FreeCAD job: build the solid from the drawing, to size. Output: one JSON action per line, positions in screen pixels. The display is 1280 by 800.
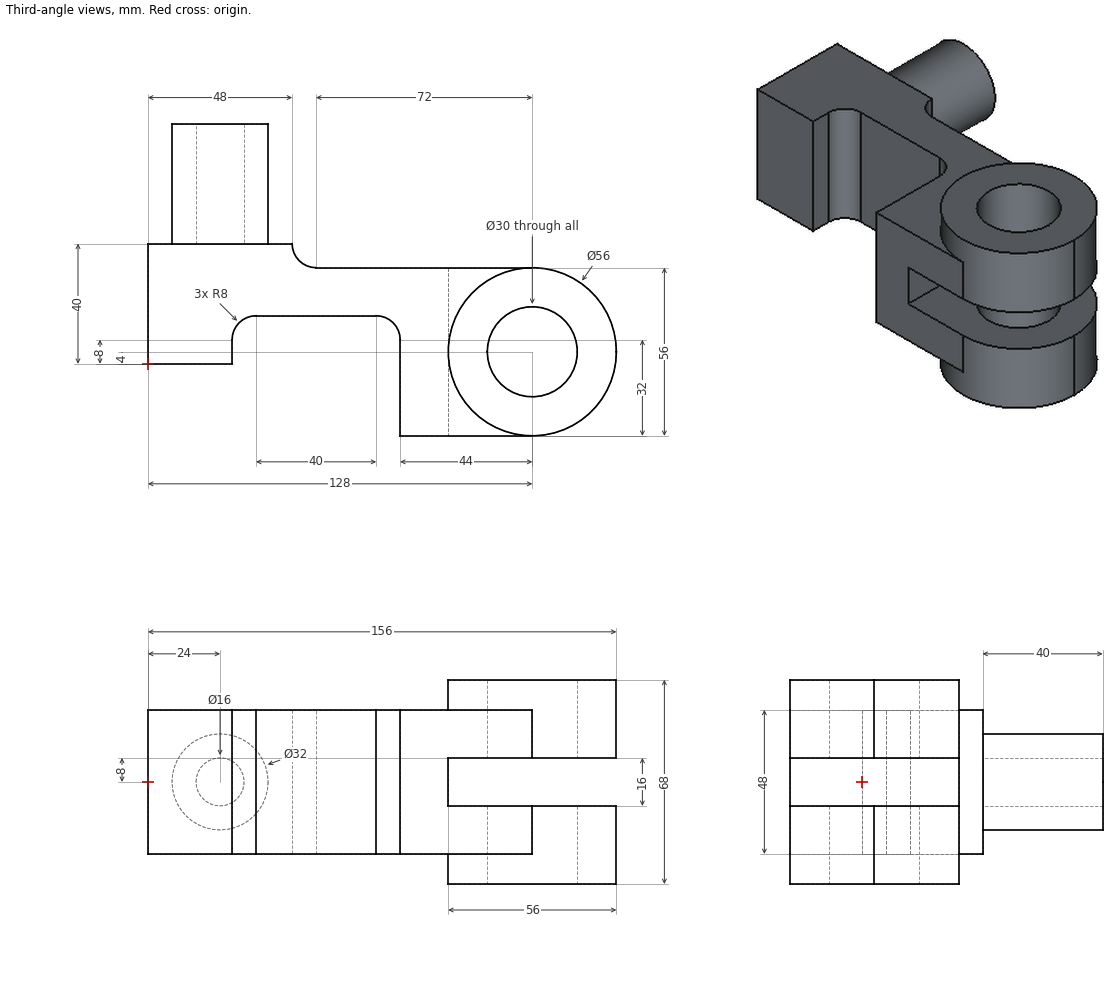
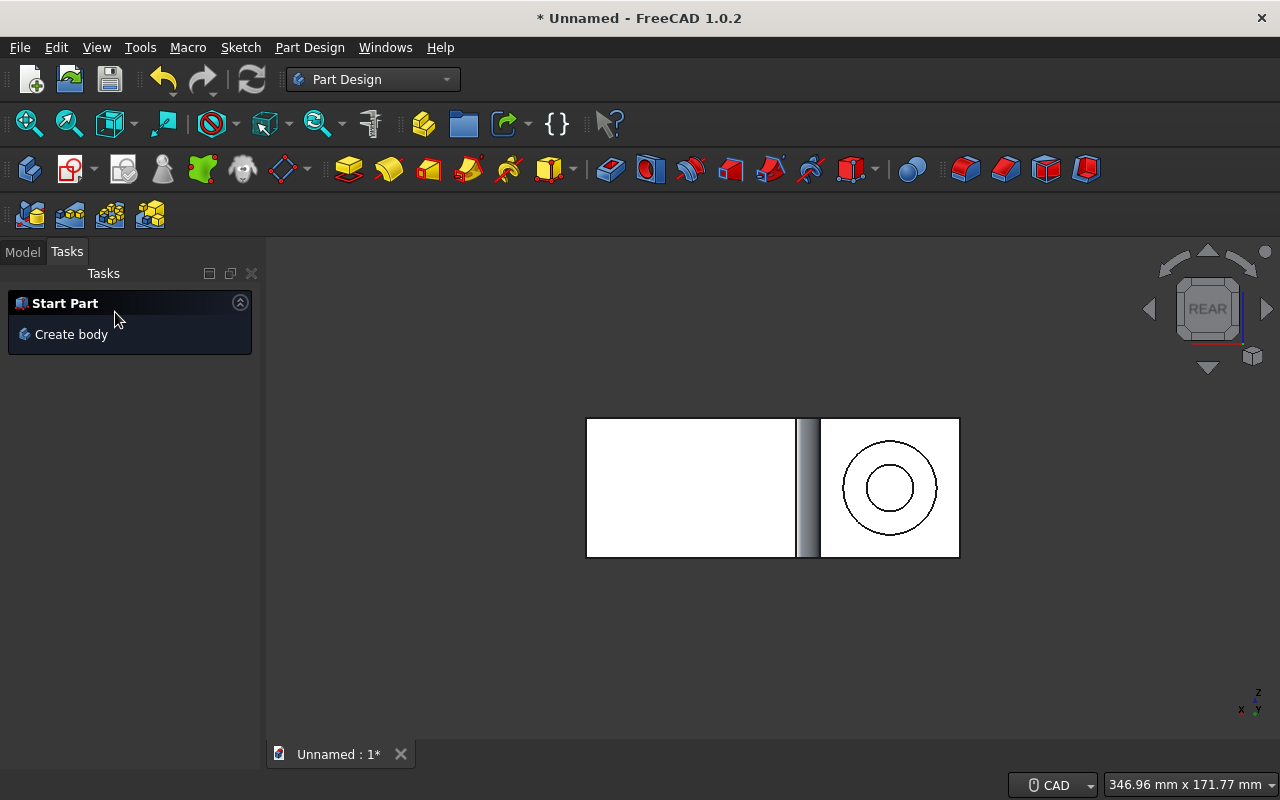
{"action": "left_click", "coordinate": [70, 170]}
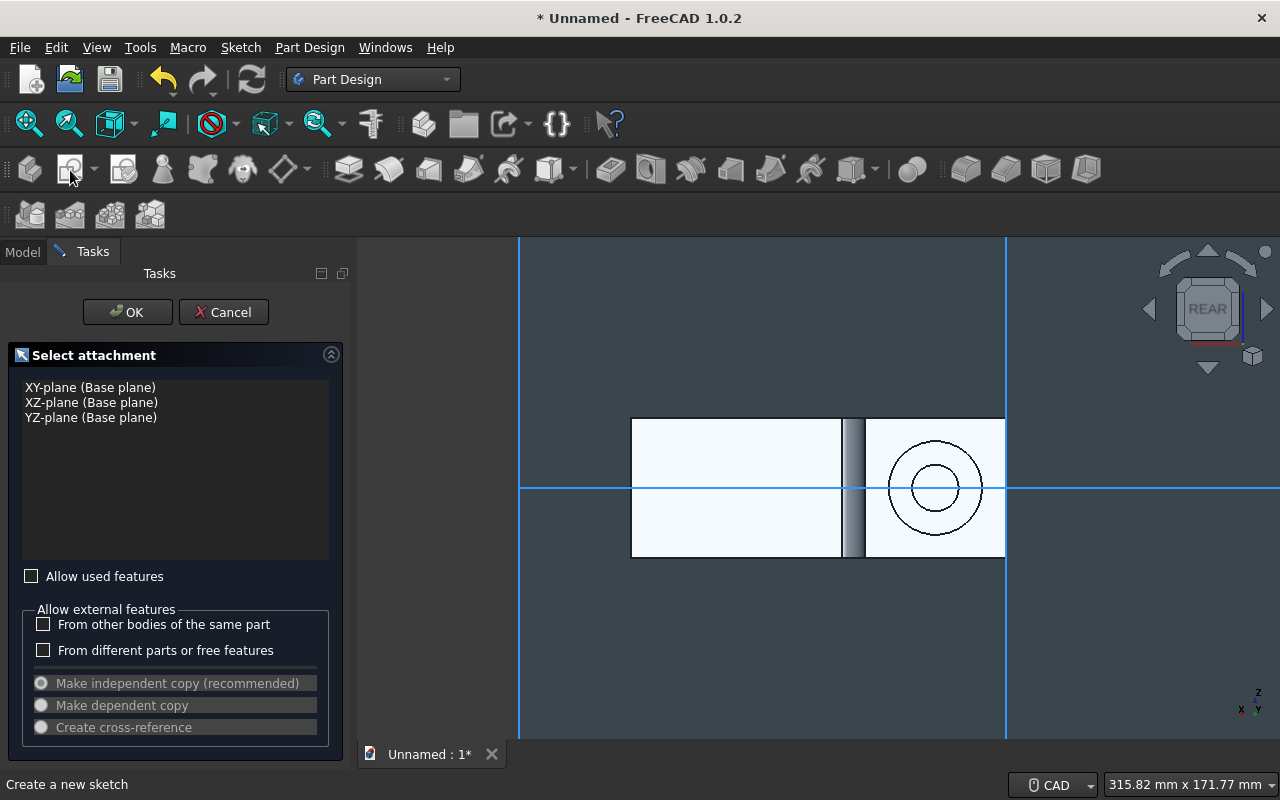
{"action": "left_click", "coordinate": [82, 388]}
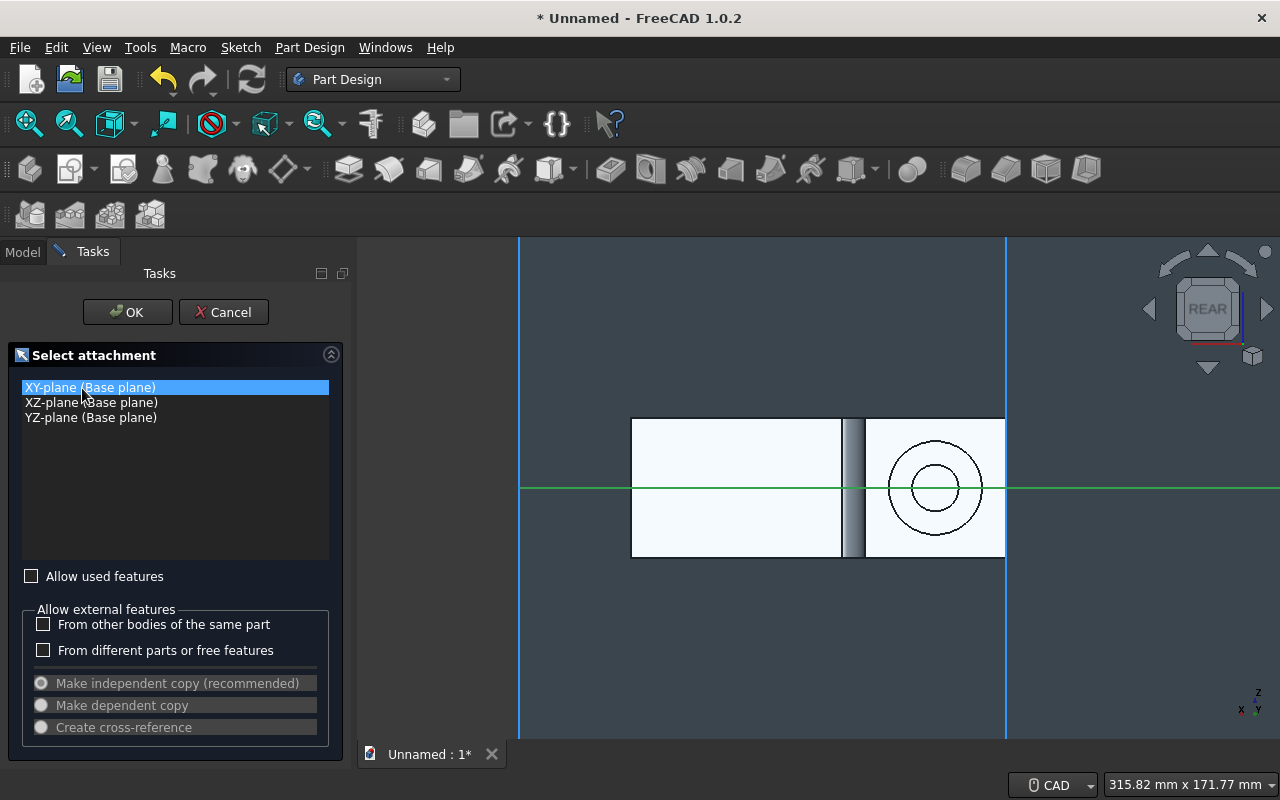
{"action": "left_click", "coordinate": [128, 312]}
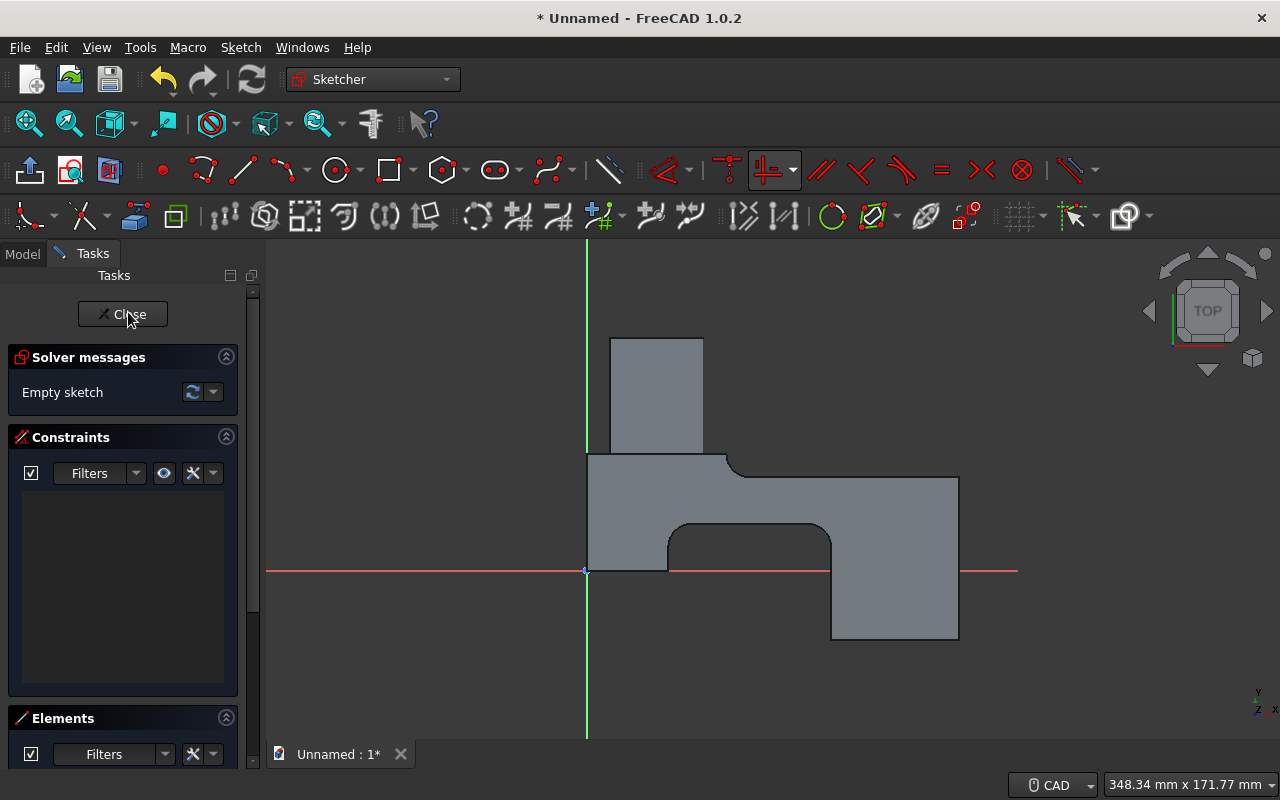
{"action": "key", "text": "q s"}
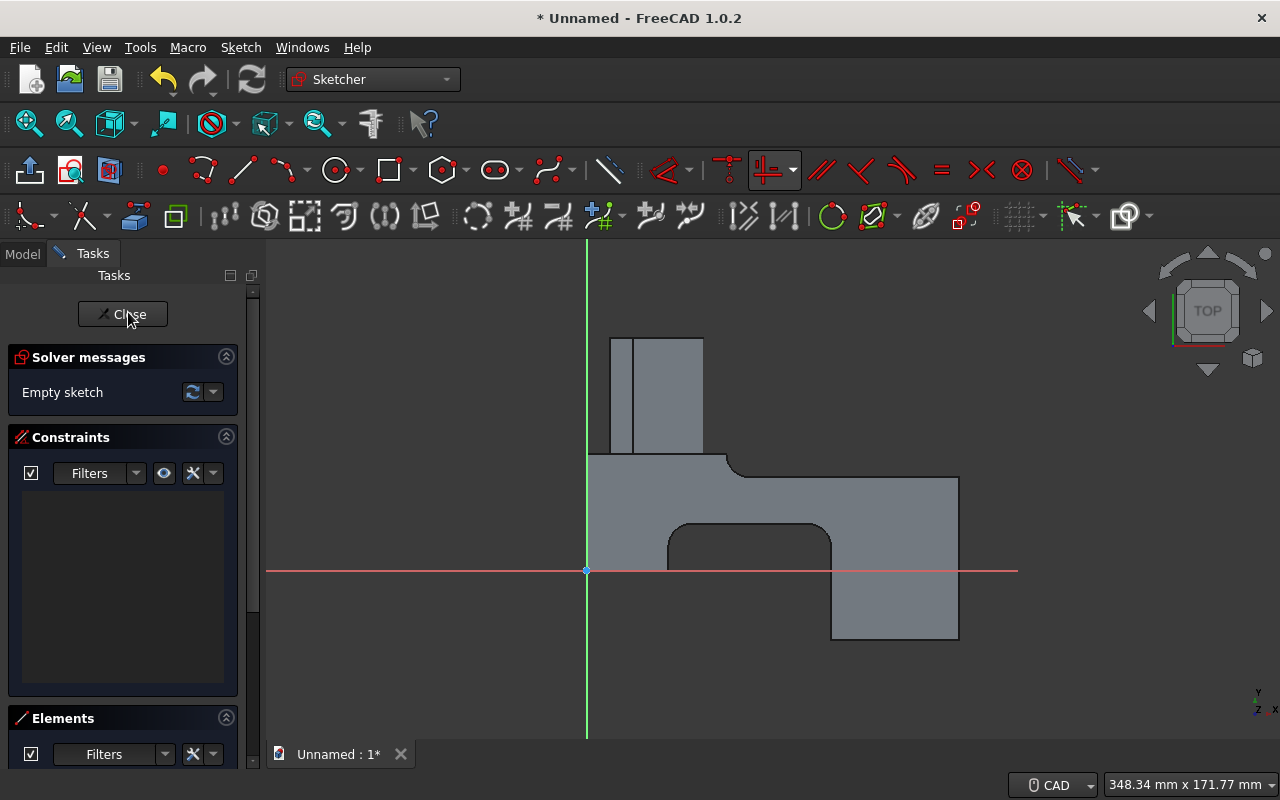
{"action": "scroll", "coordinate": [1115, 644], "scroll_direction": "up", "scroll_amount": 3}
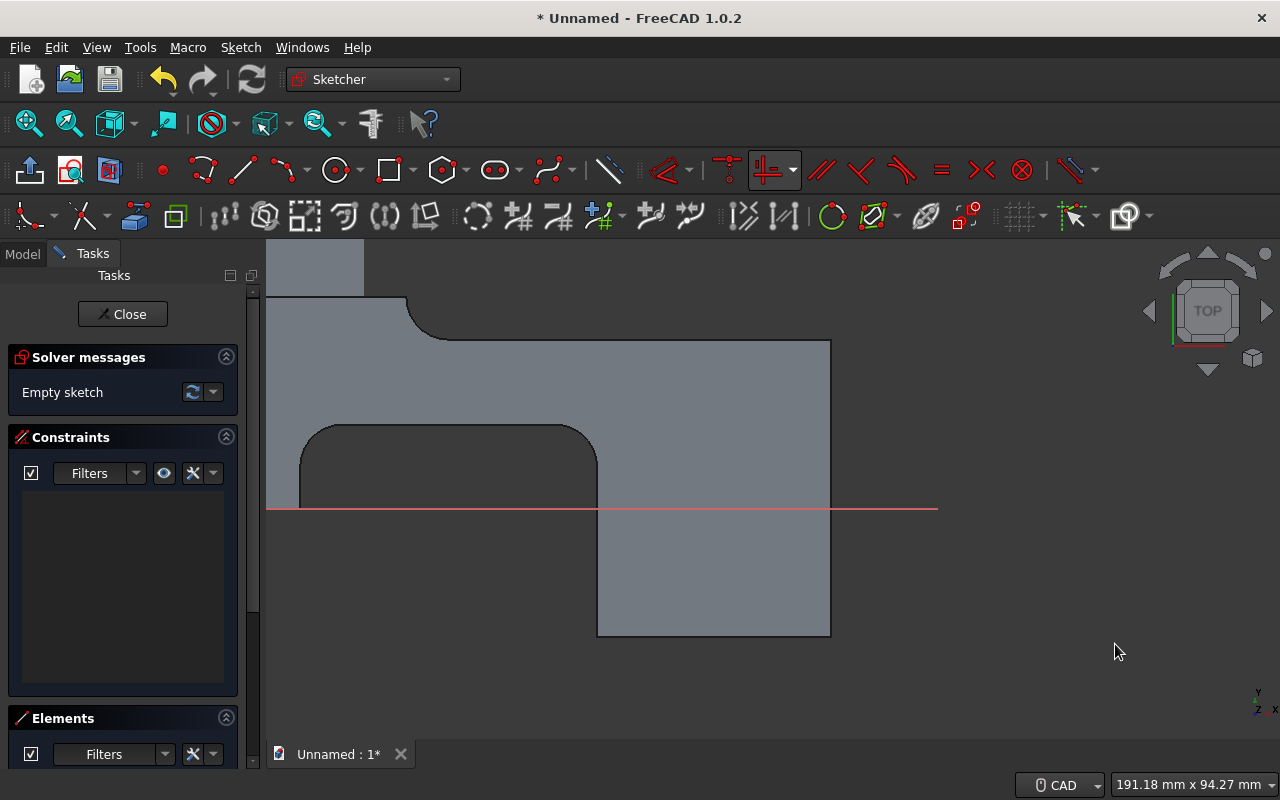
{"action": "key", "text": "g c"}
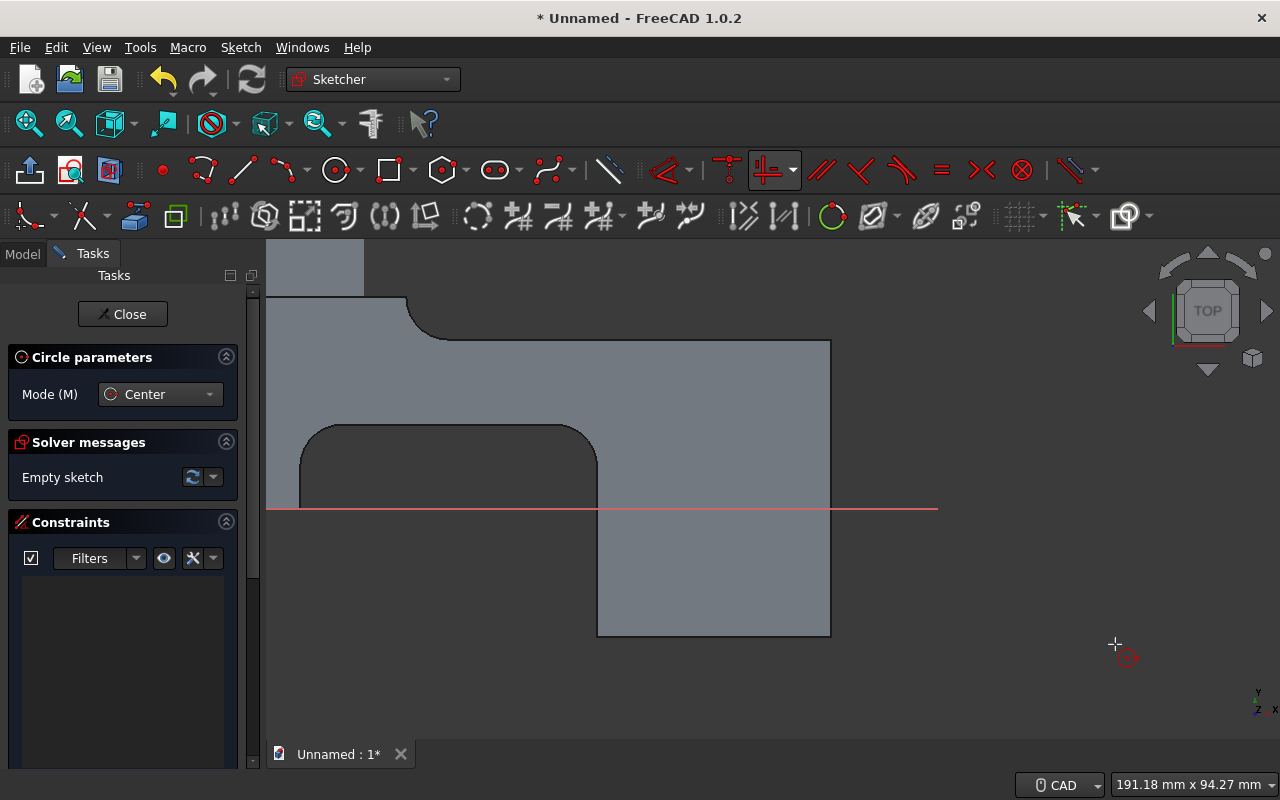
{"action": "left_click", "coordinate": [831, 488]}
{"action": "mouse_move", "coordinate": [936, 383]}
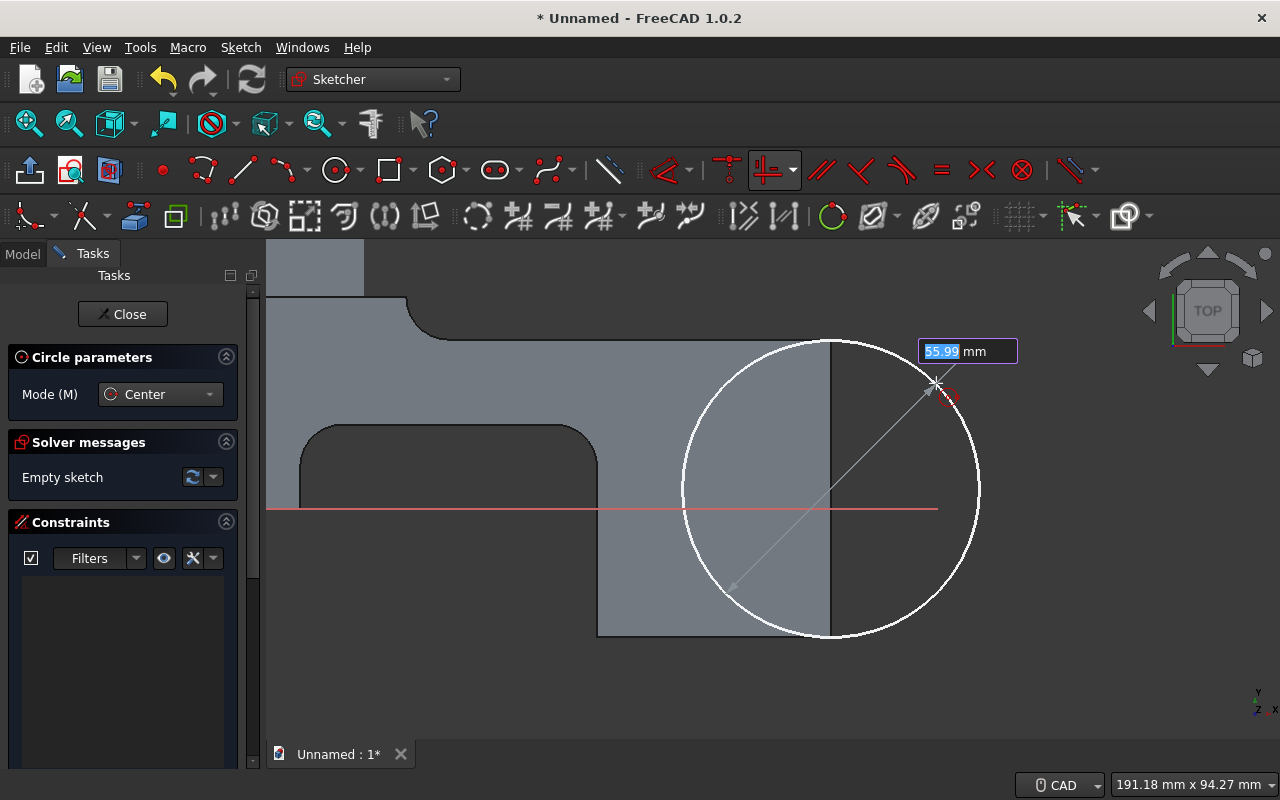
{"action": "type", "text": "56"}
{"action": "key", "text": "Return"}
{"action": "key", "text": "Escape"}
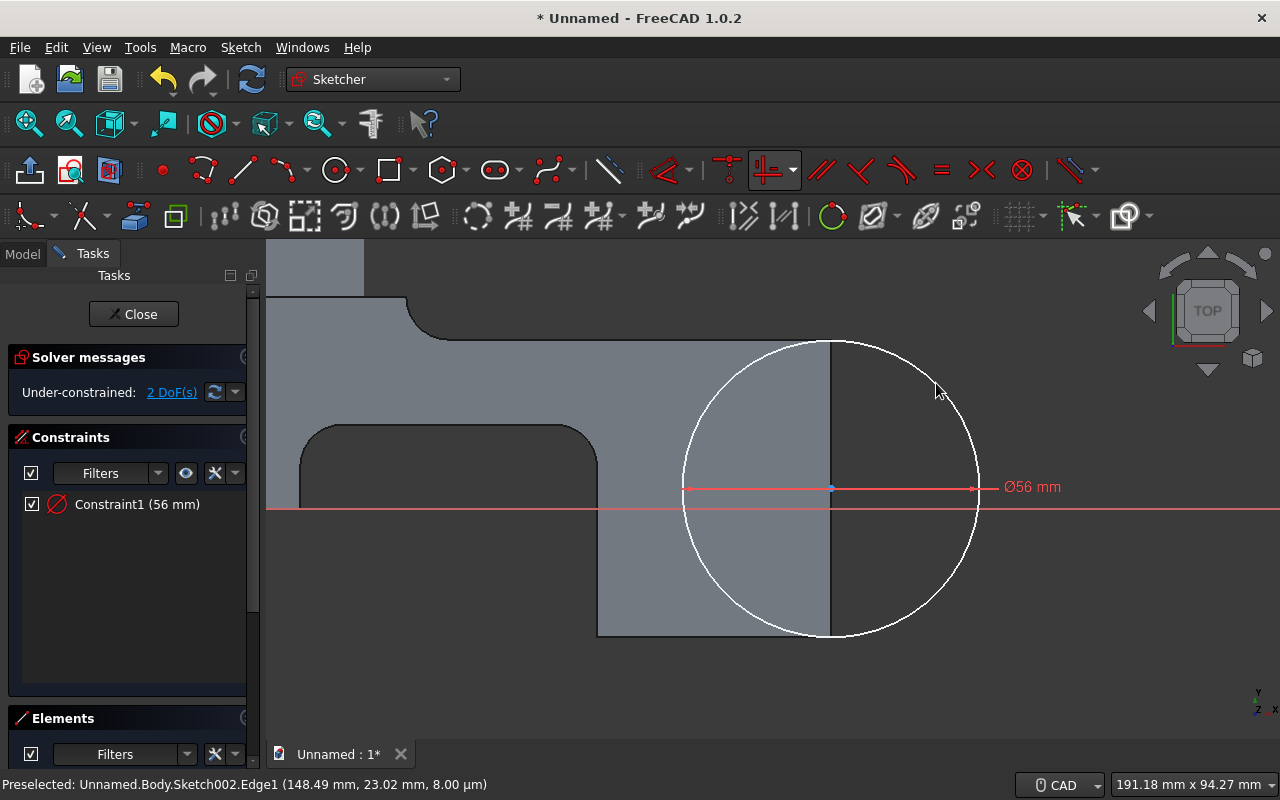
{"action": "key", "text": "d"}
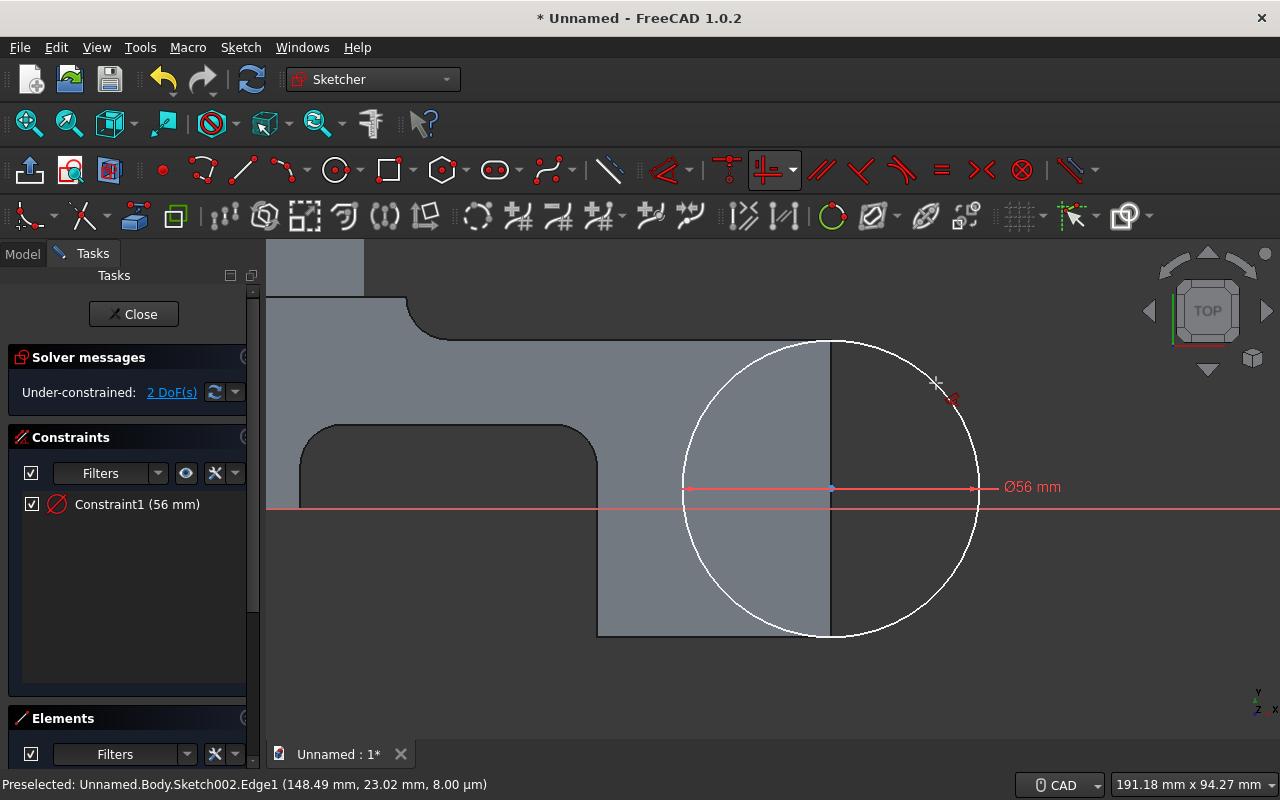
{"action": "scroll", "coordinate": [831, 489], "scroll_direction": "up", "scroll_amount": 4}